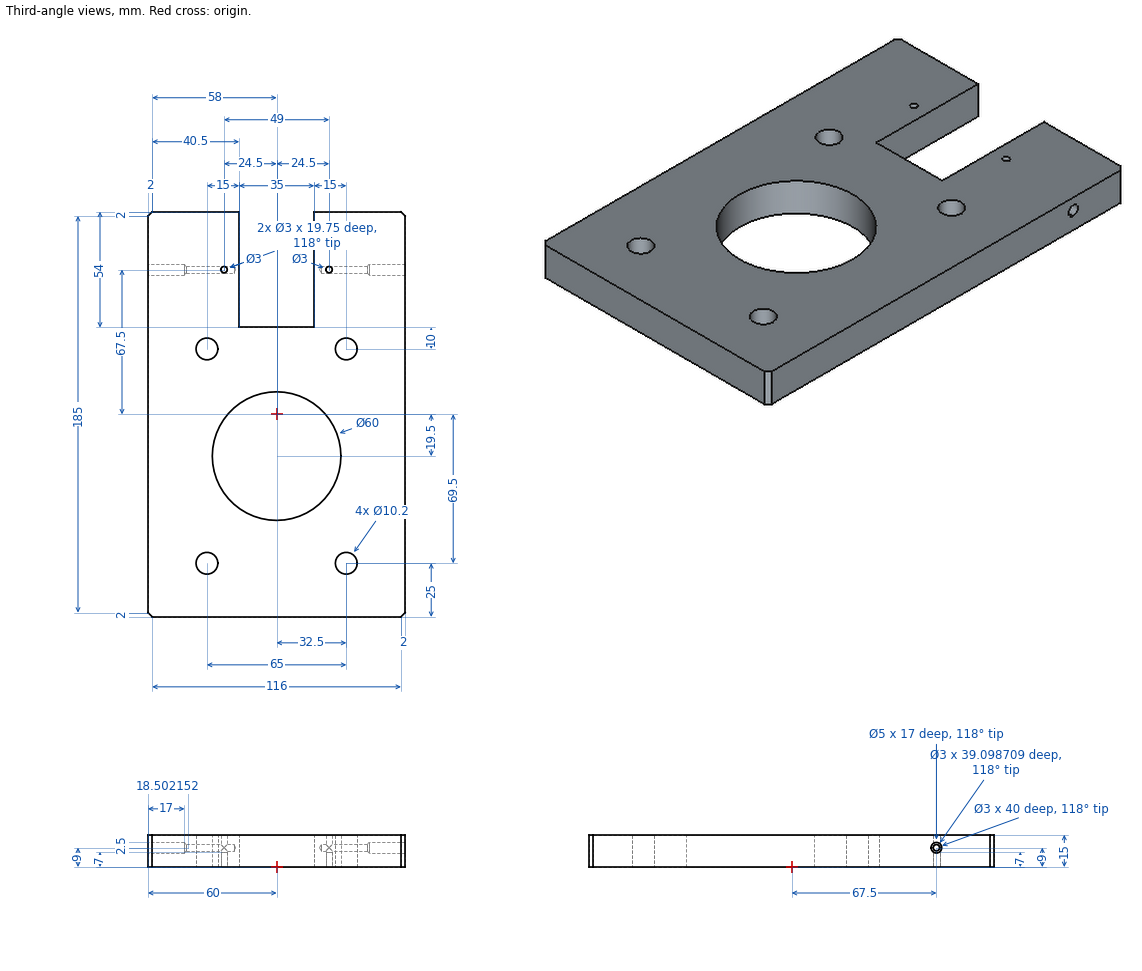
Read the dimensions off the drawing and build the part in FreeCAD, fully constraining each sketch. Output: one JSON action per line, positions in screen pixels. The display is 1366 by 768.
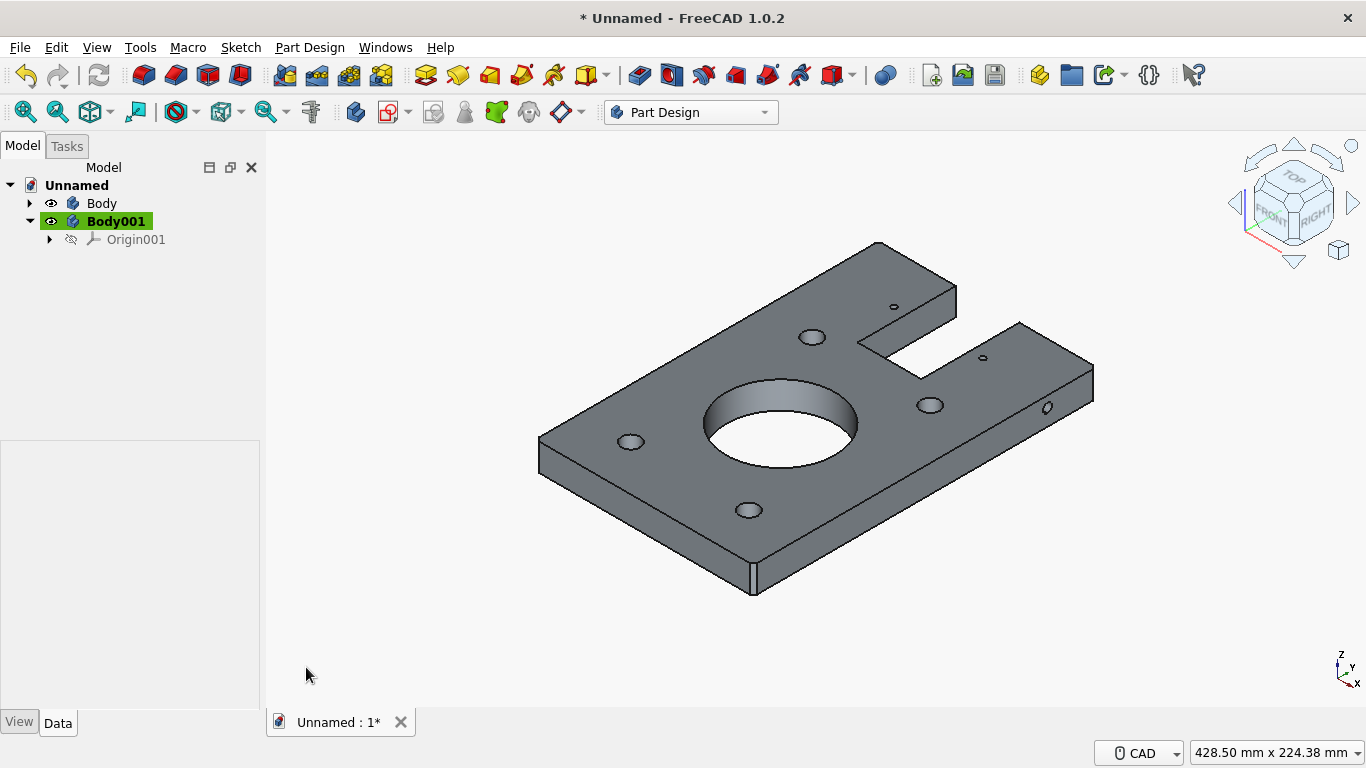
{"action": "left_click", "coordinate": [388, 112]}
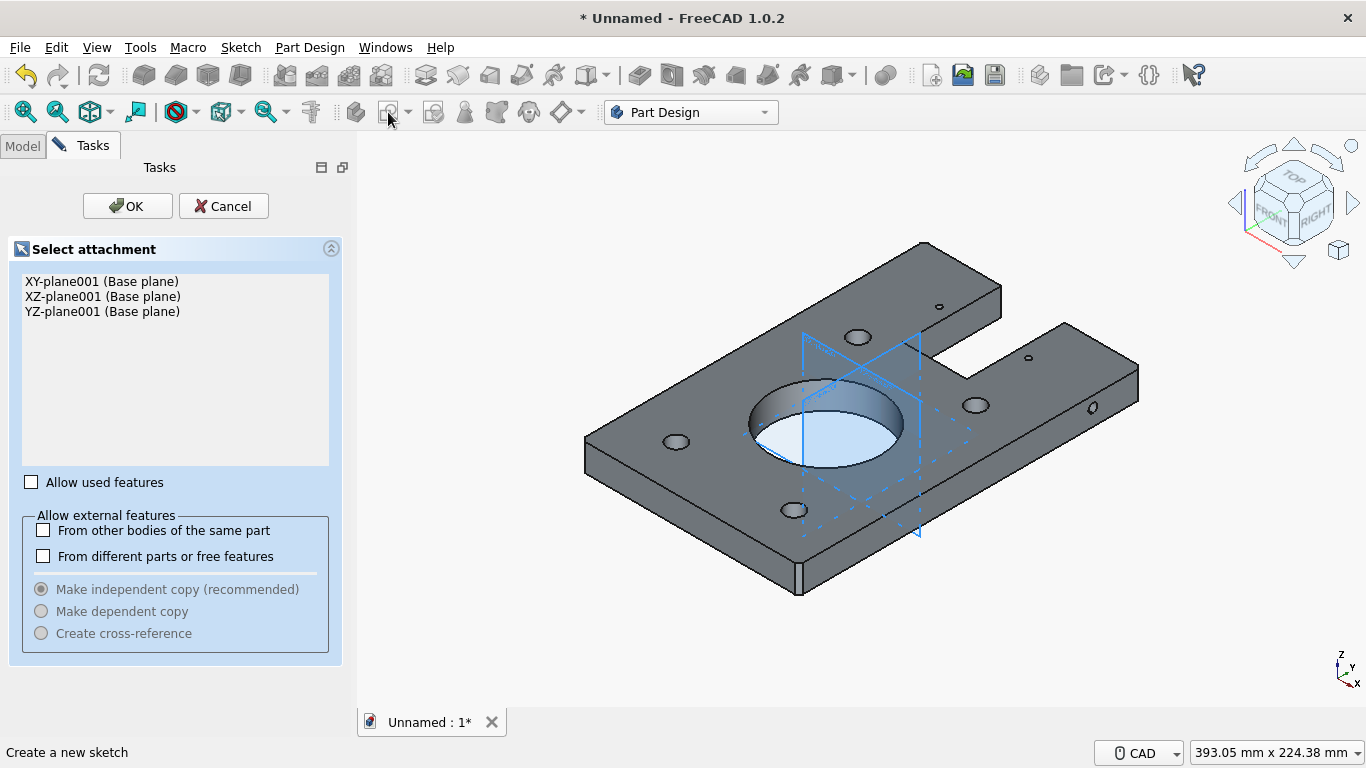
{"action": "left_click", "coordinate": [82, 282]}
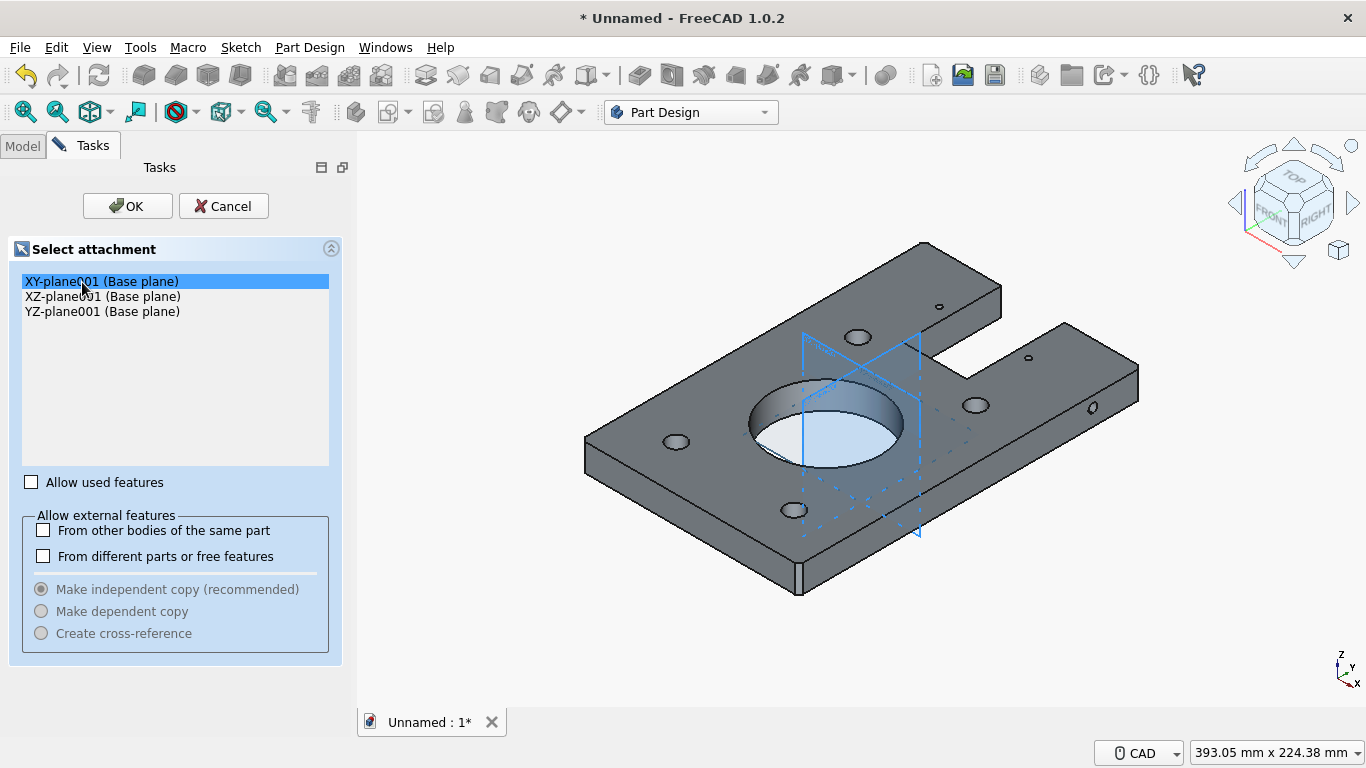
{"action": "left_click", "coordinate": [128, 206]}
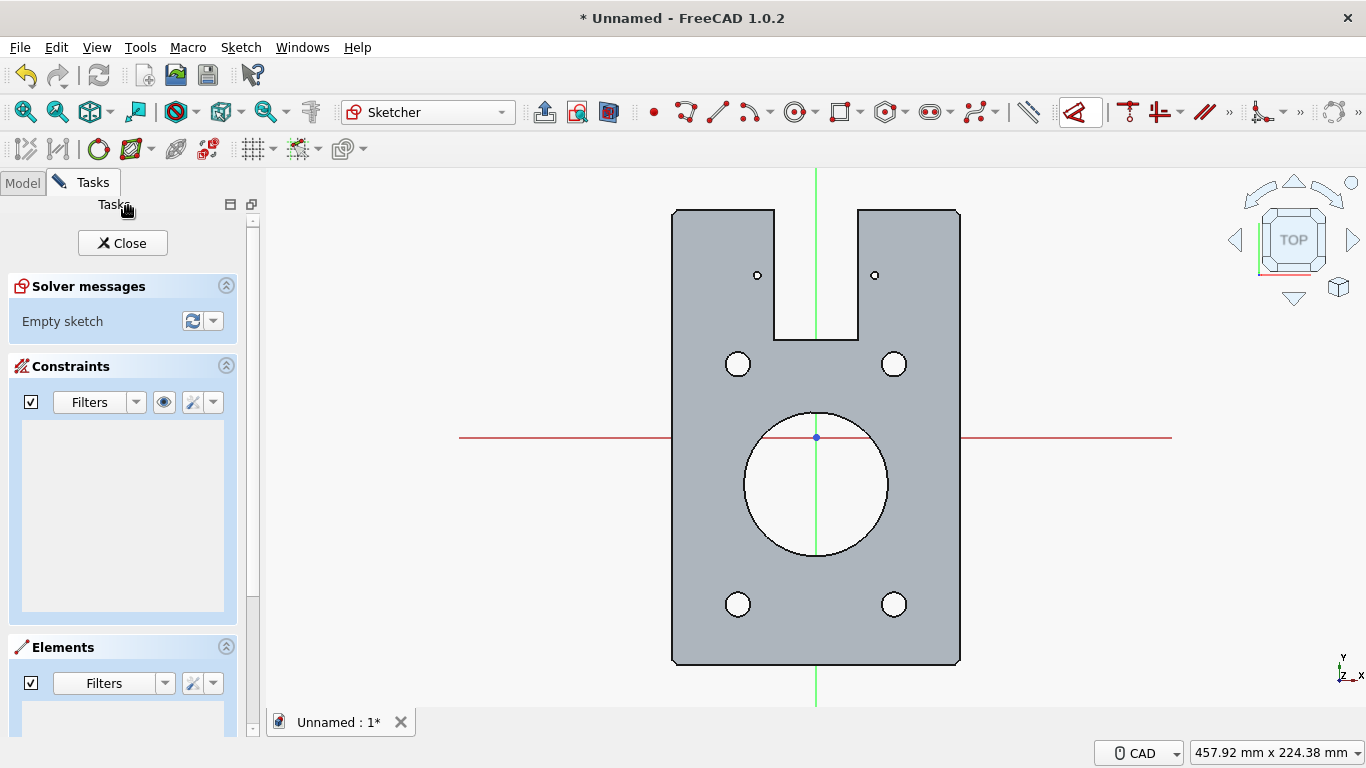
{"action": "scroll", "coordinate": [758, 267], "scroll_direction": "up", "scroll_amount": 15}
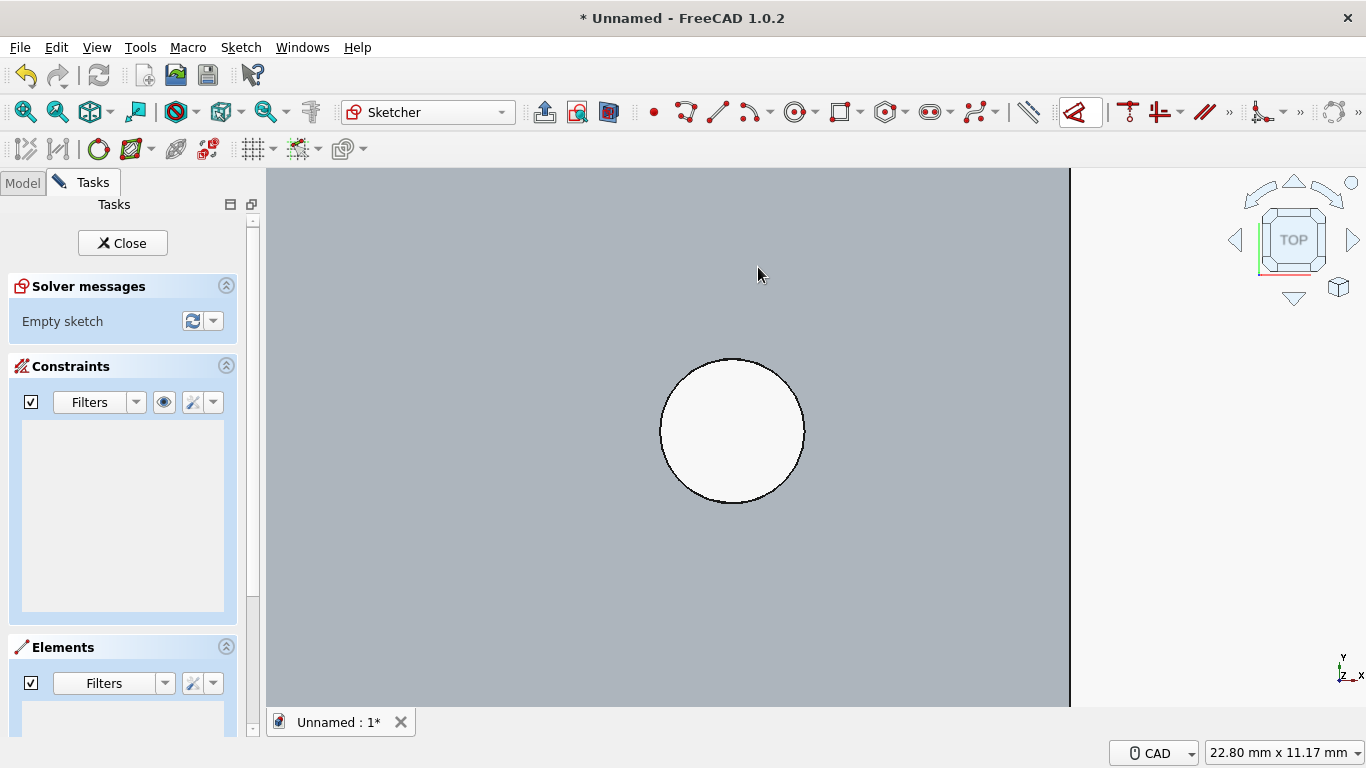
{"action": "scroll", "coordinate": [720, 426], "scroll_direction": "up", "scroll_amount": 4}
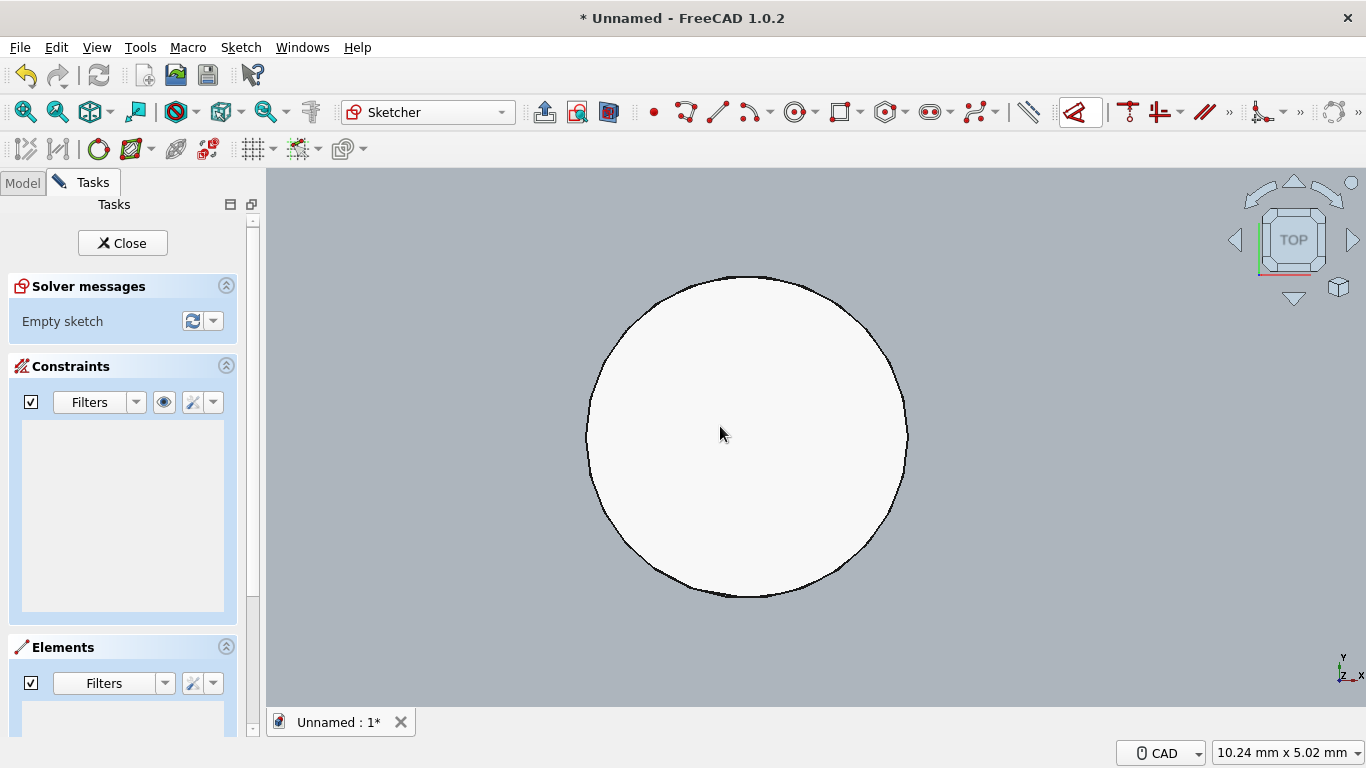
{"action": "left_click", "coordinate": [796, 112]}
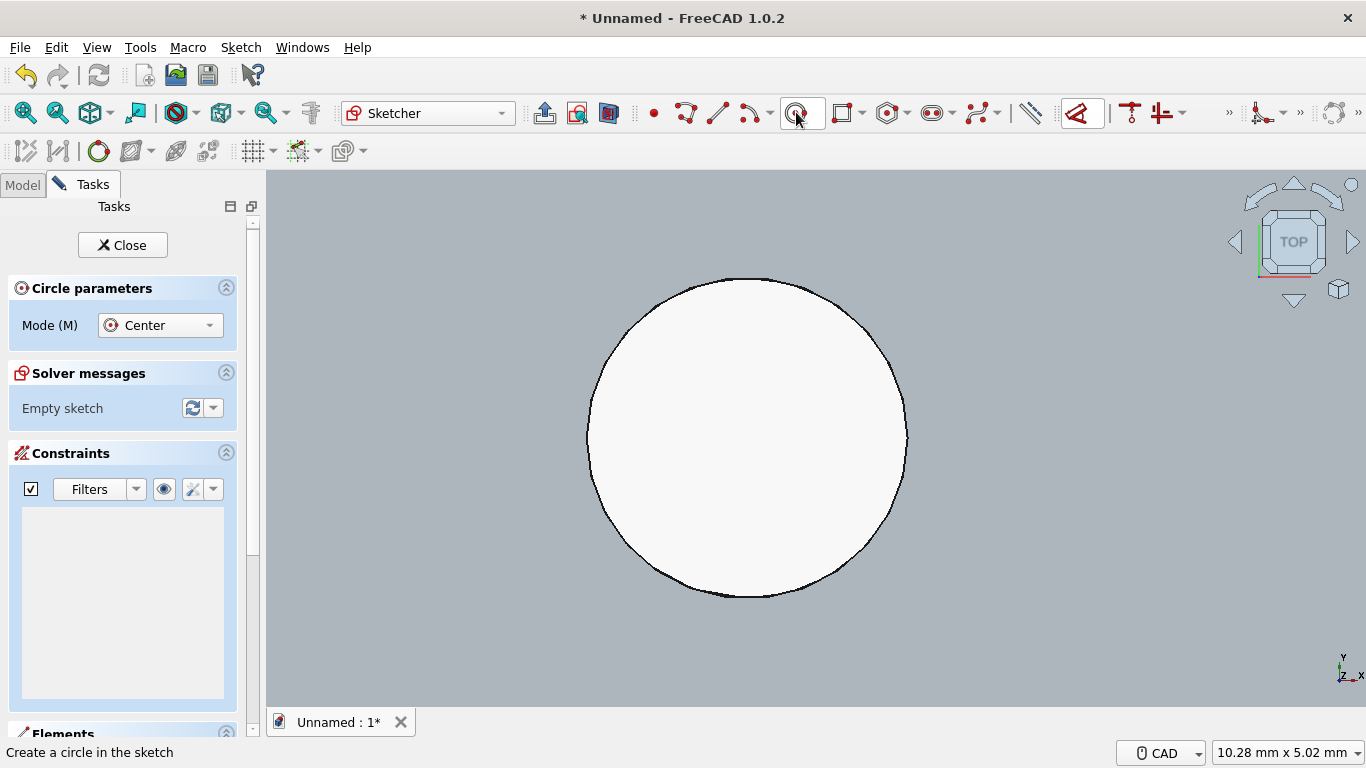
{"action": "left_click", "coordinate": [747, 438]}
{"action": "mouse_move", "coordinate": [861, 325]}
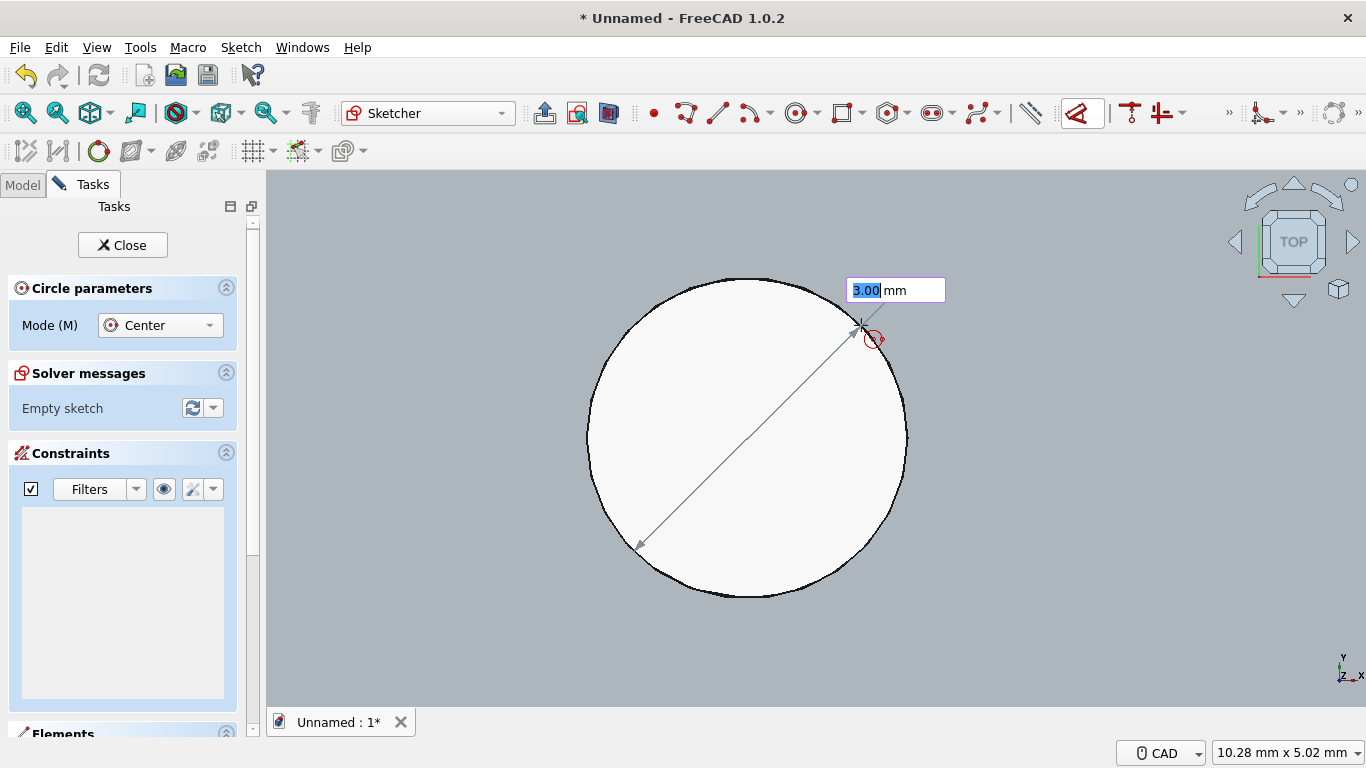
{"action": "type", "text": "3"}
{"action": "key", "text": "Return"}
{"action": "key", "text": "Escape"}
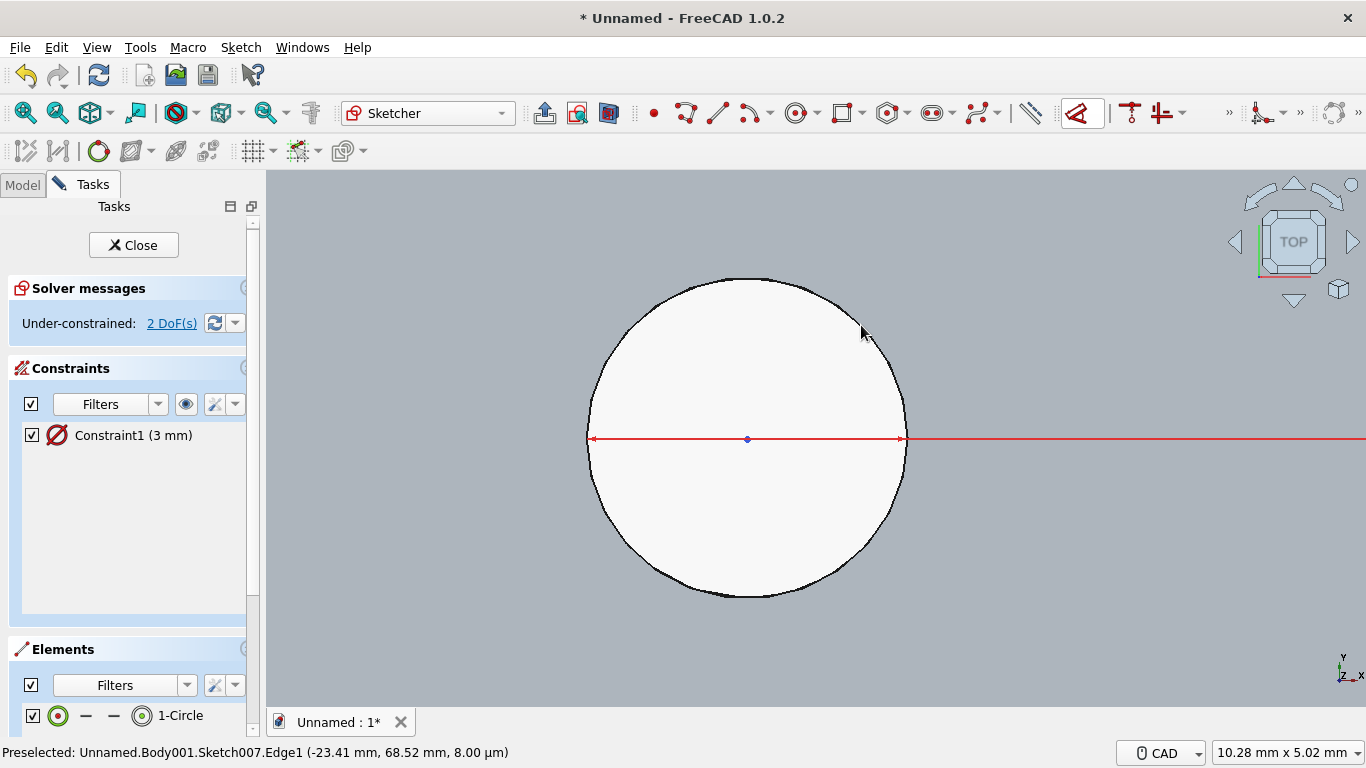
{"action": "left_click", "coordinate": [747, 439]}